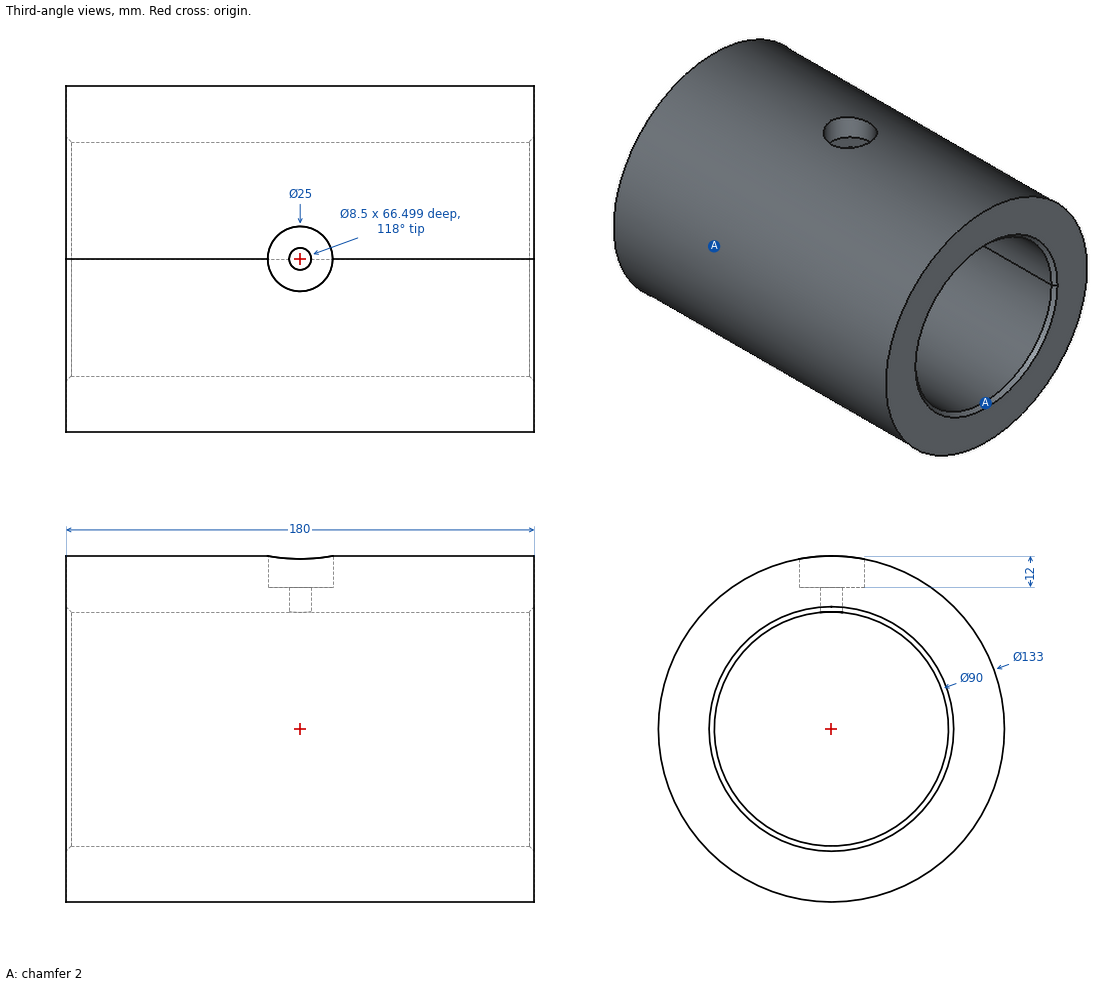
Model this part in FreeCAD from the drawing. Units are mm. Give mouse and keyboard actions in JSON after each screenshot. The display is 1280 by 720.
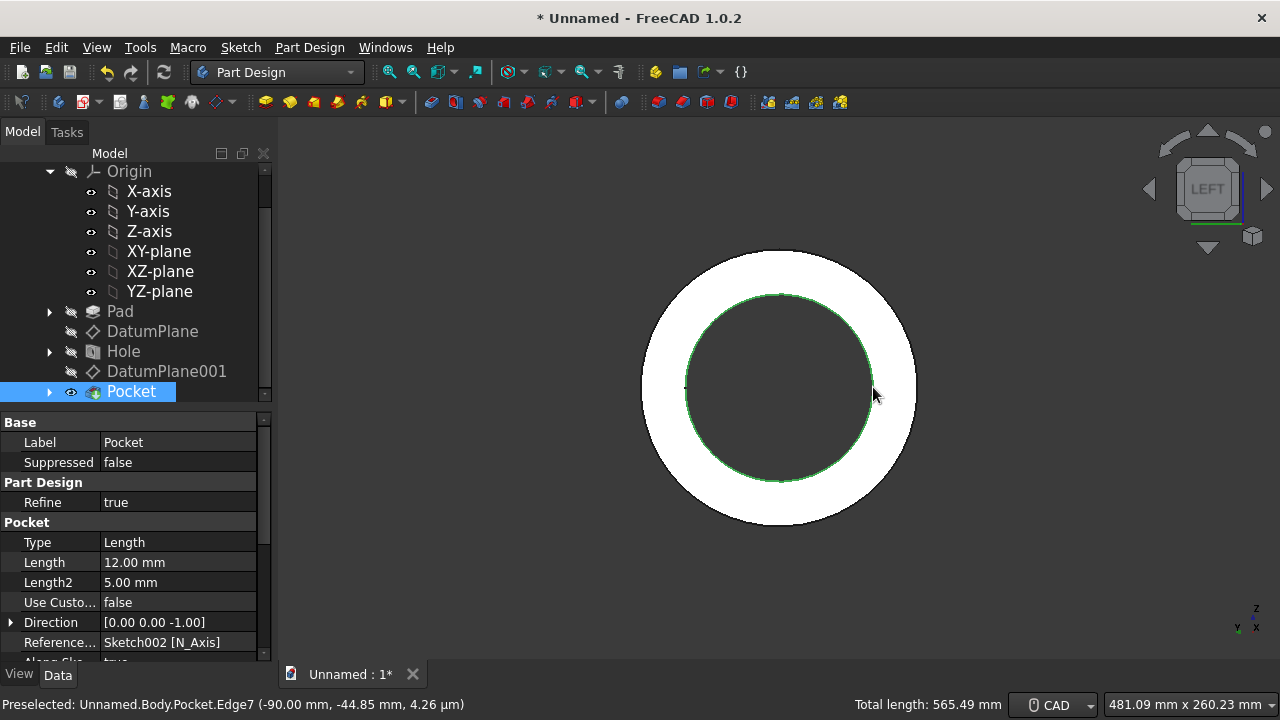
{"action": "left_click", "coordinate": [684, 102]}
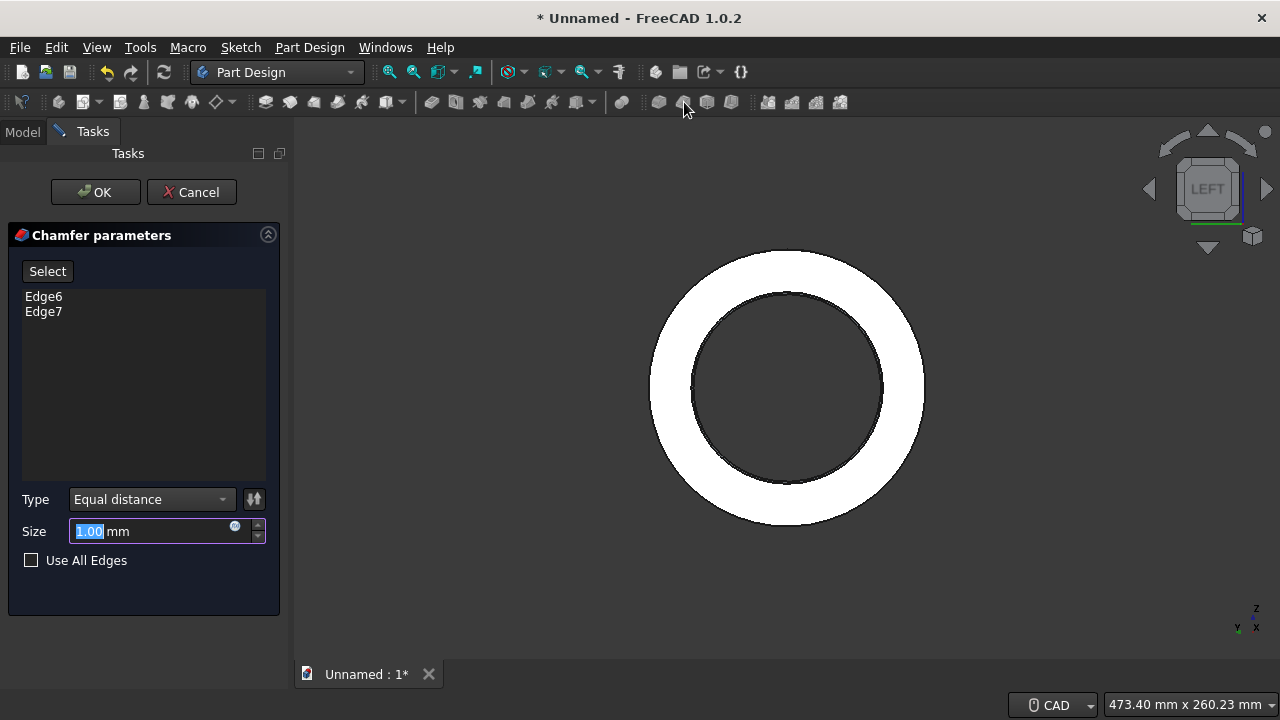
{"action": "type", "text": "2"}
{"action": "key", "text": "Tab"}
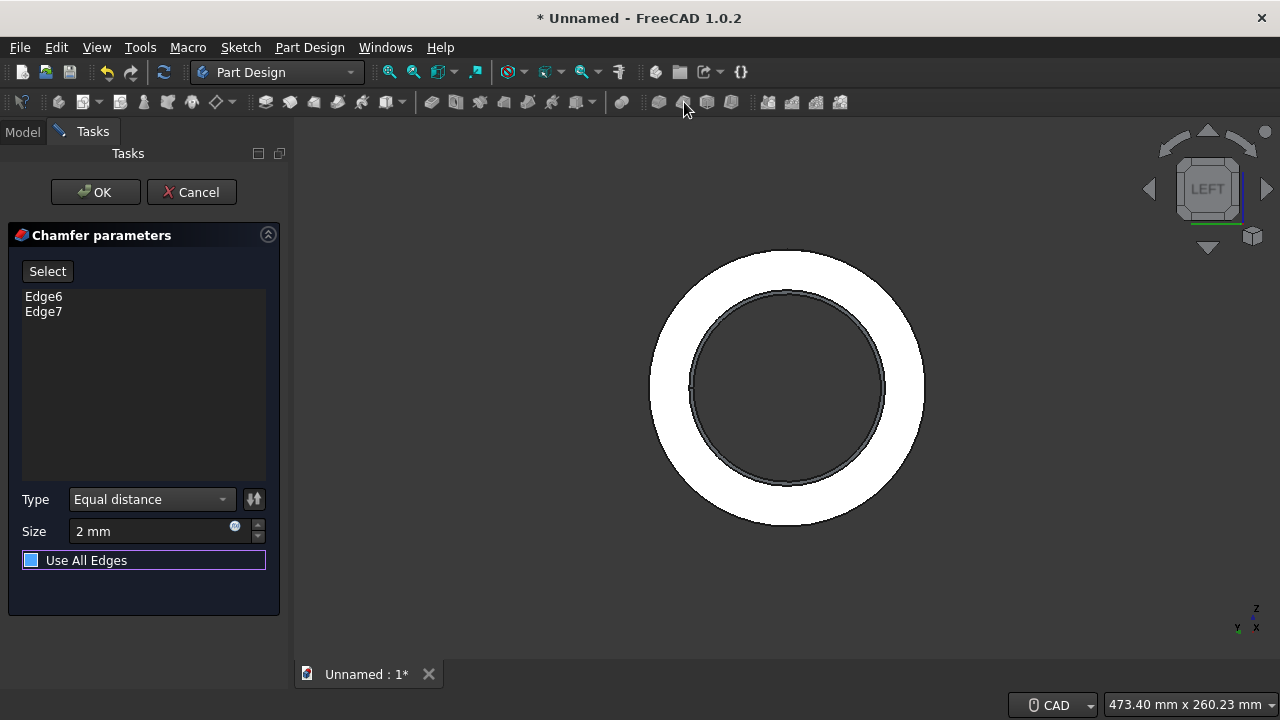
{"action": "left_click", "coordinate": [96, 192]}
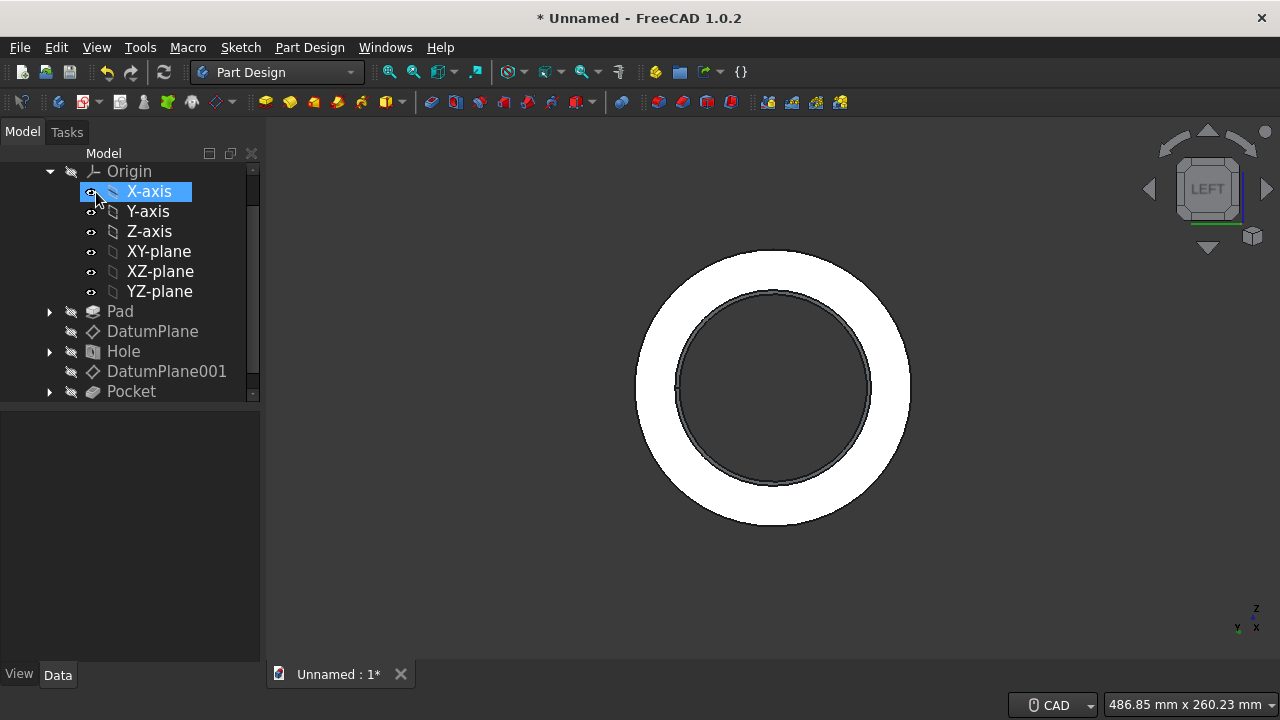
{"action": "key", "text": "0"}